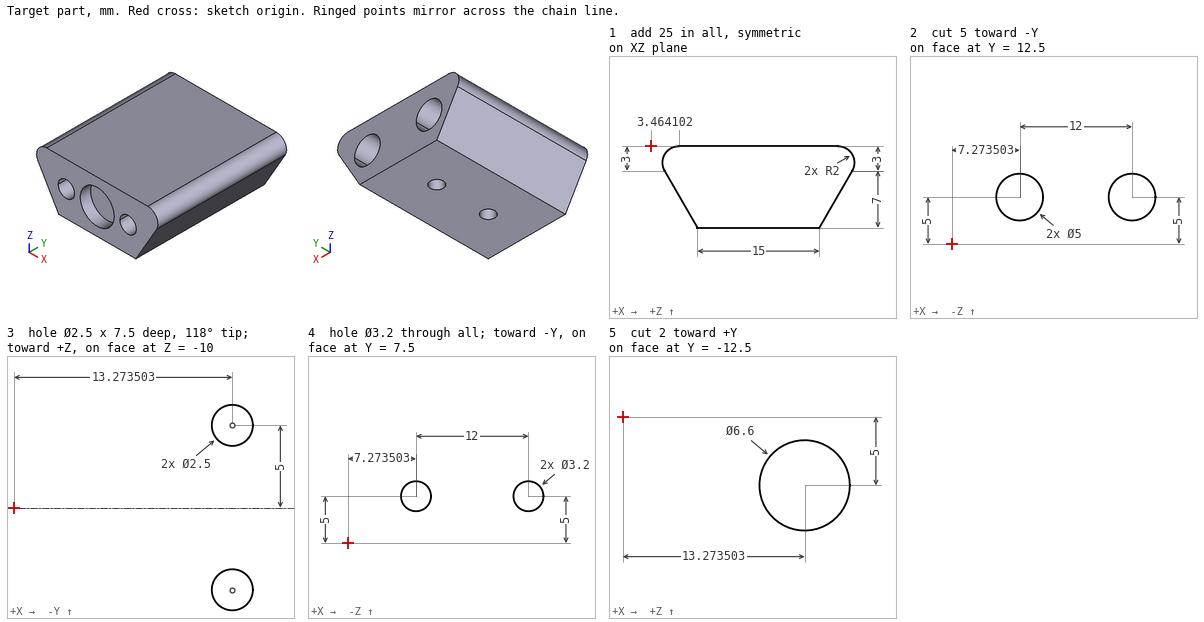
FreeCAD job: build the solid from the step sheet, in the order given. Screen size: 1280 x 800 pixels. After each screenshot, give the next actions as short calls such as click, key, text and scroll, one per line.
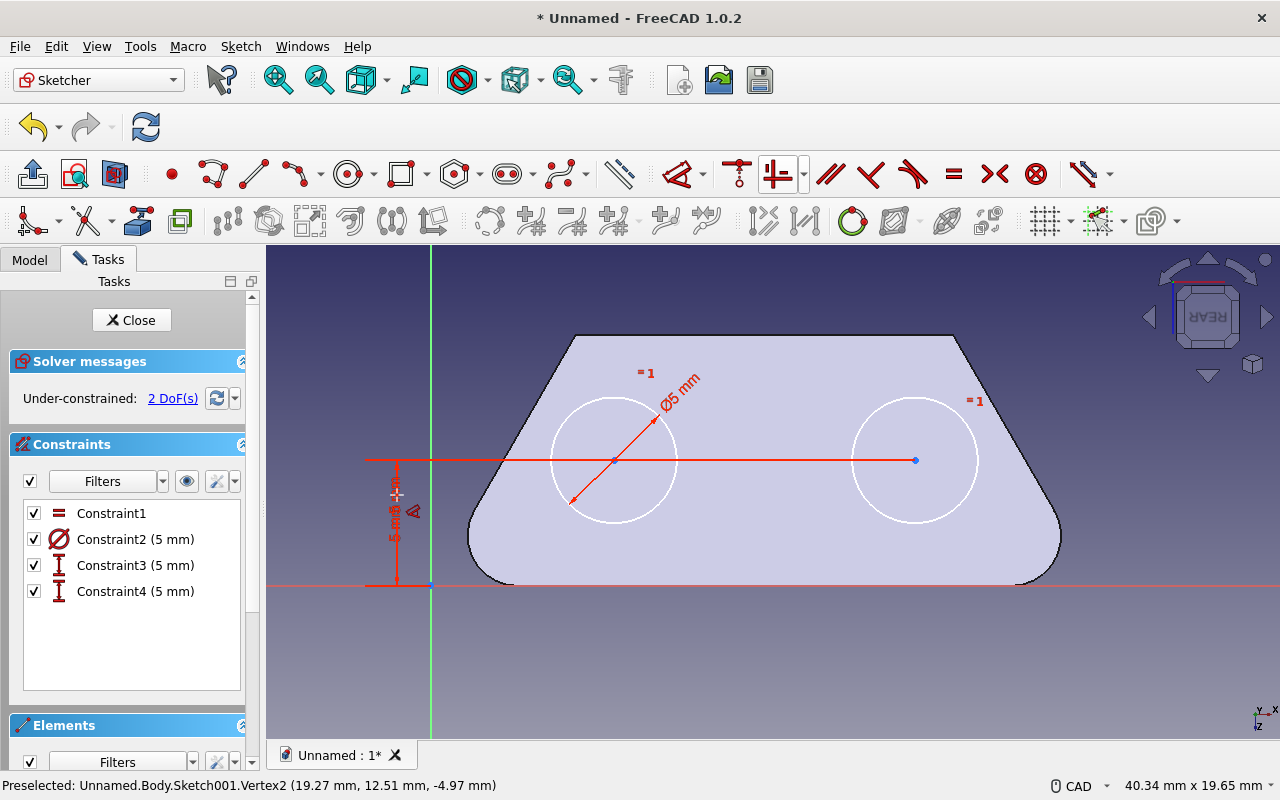
click(614, 460)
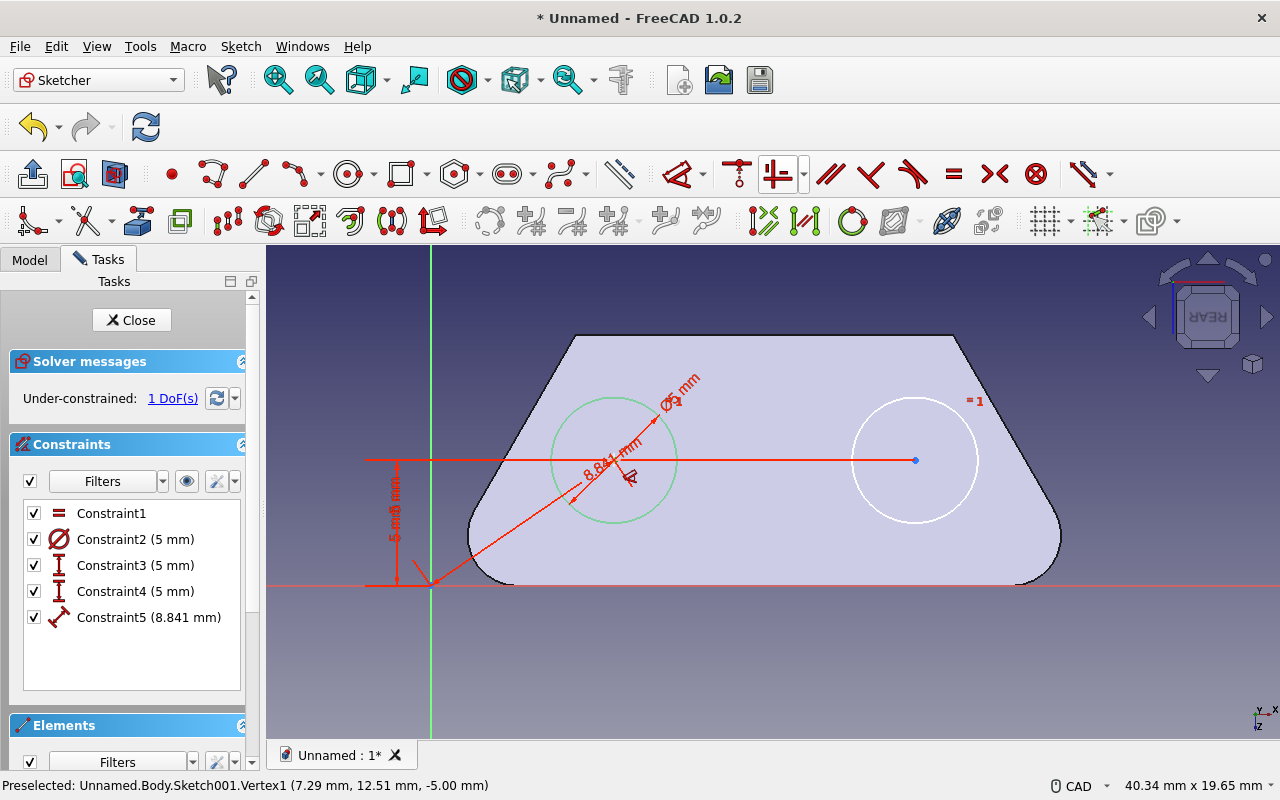
click(915, 460)
click(764, 426)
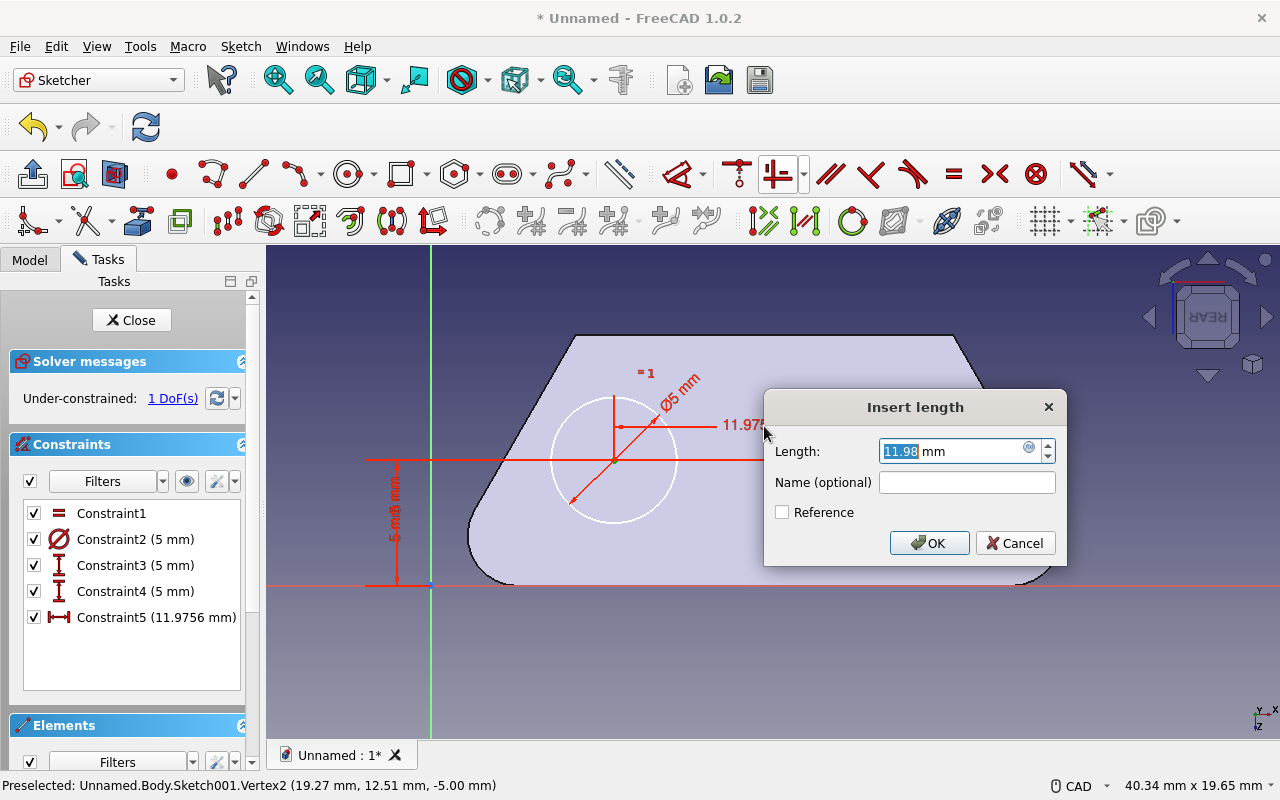
text(12)
key(Return)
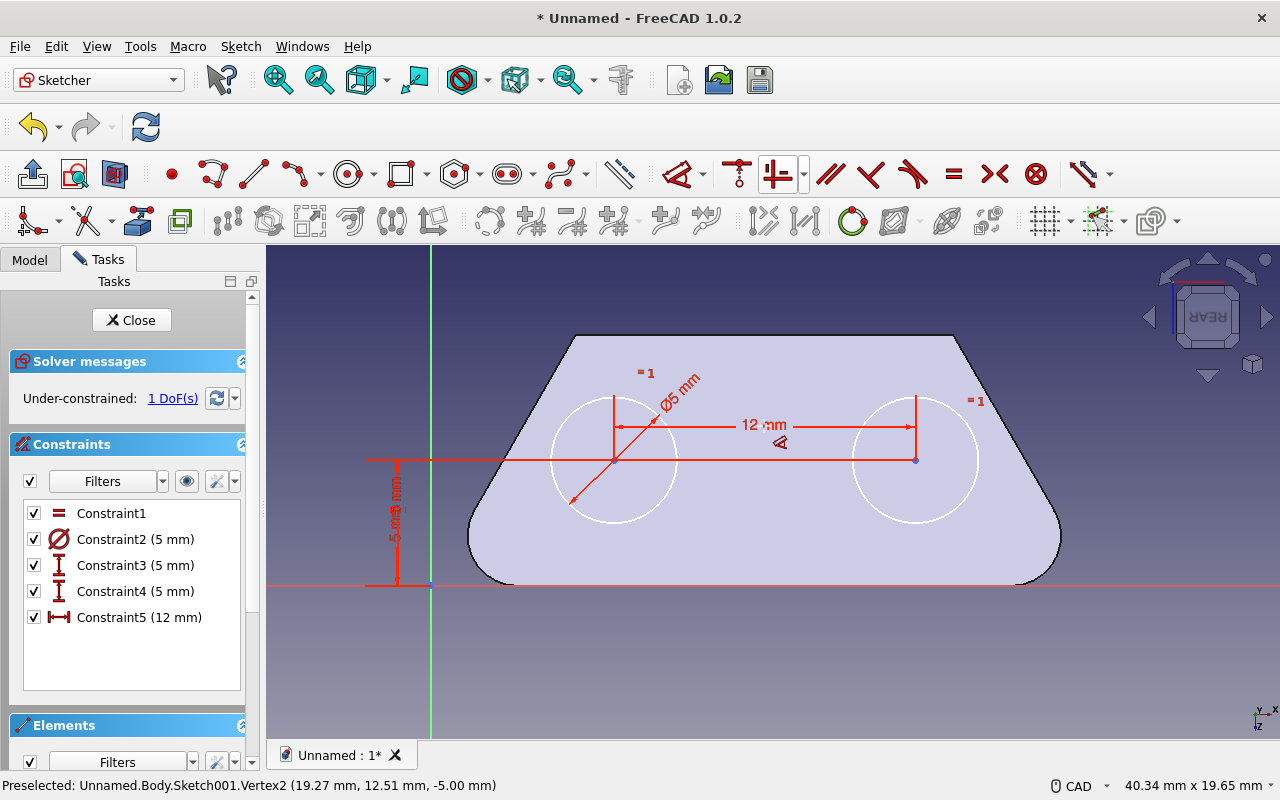
click(614, 460)
click(522, 620)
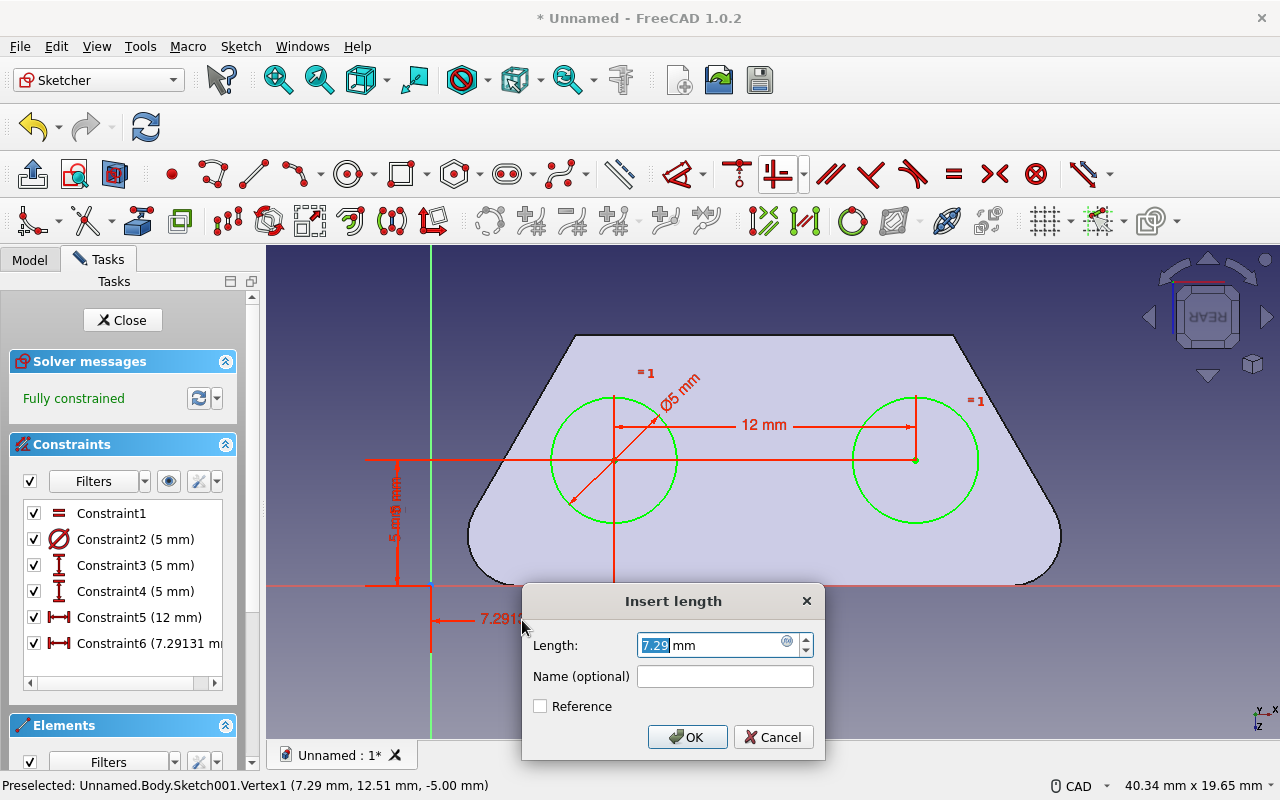
text(7.273503)
key(Return)
key(Escape)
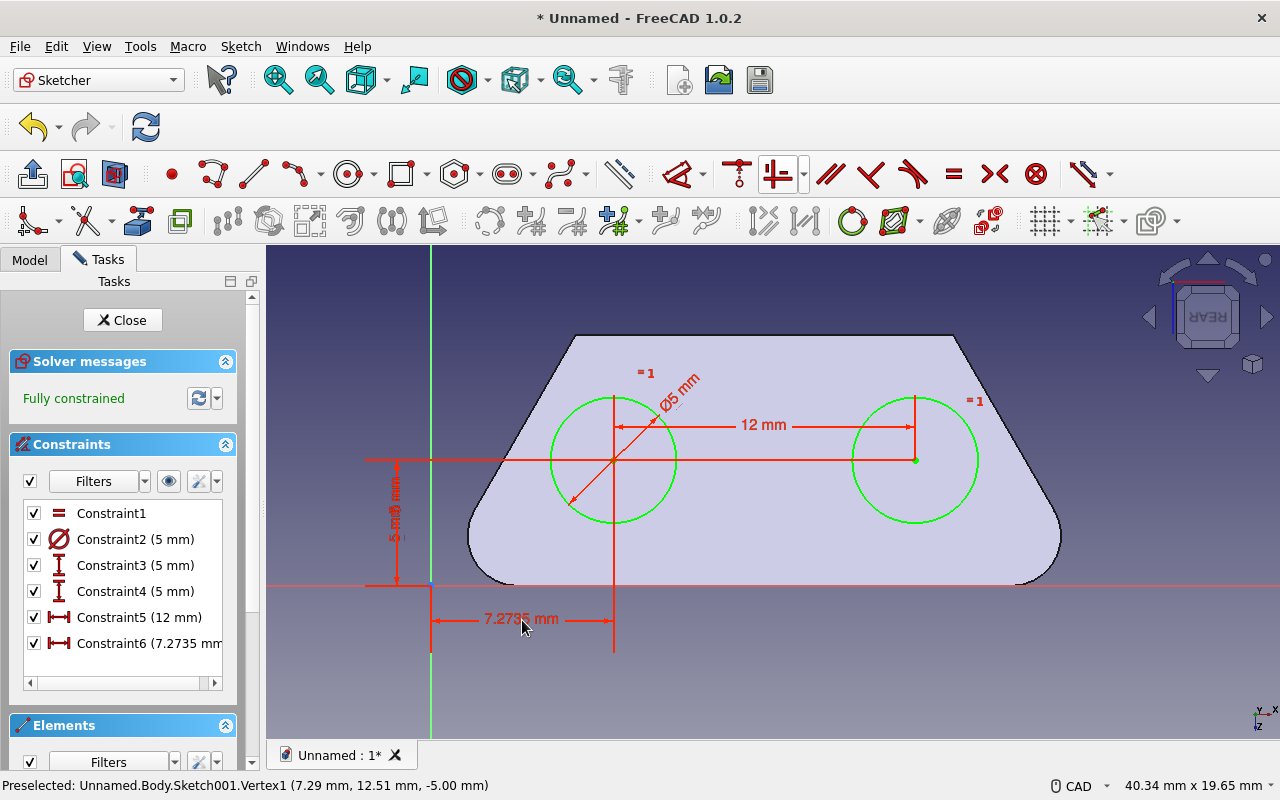
click(123, 320)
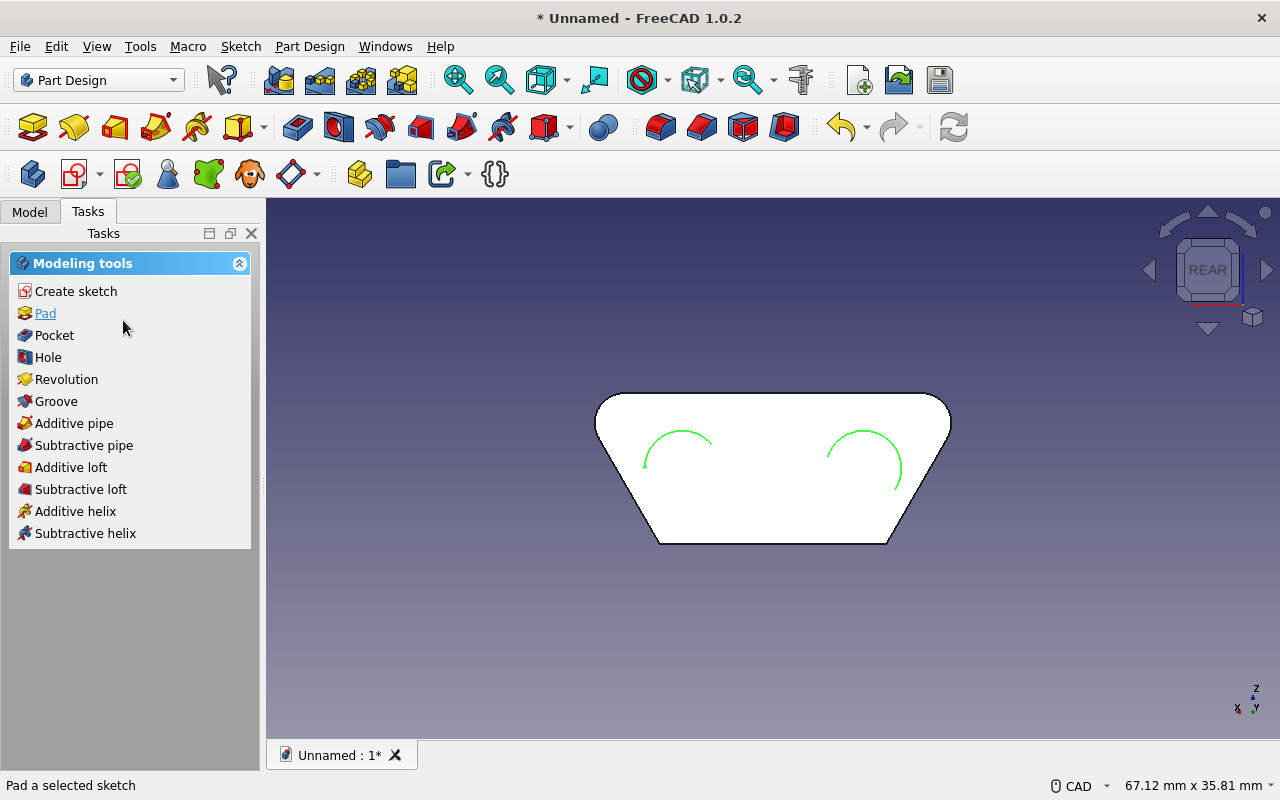
click(298, 128)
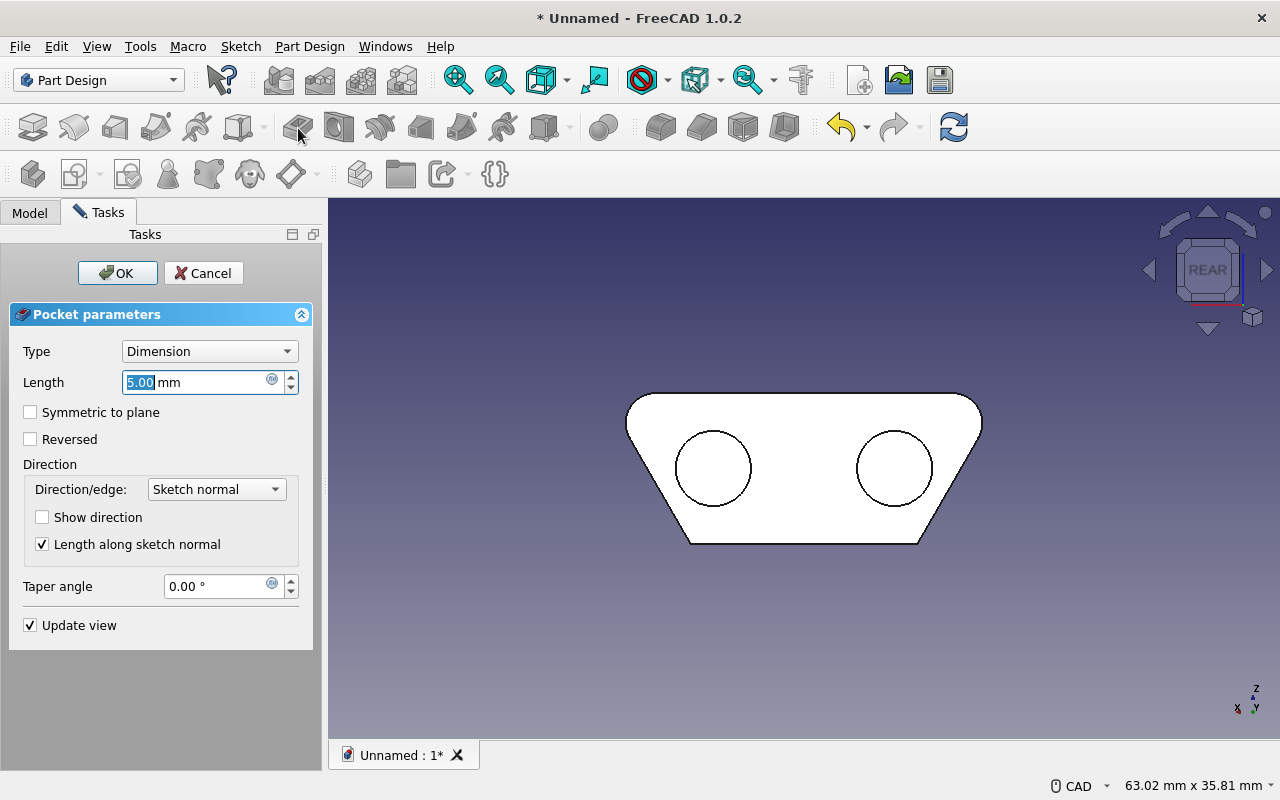
text(5)
key(Tab)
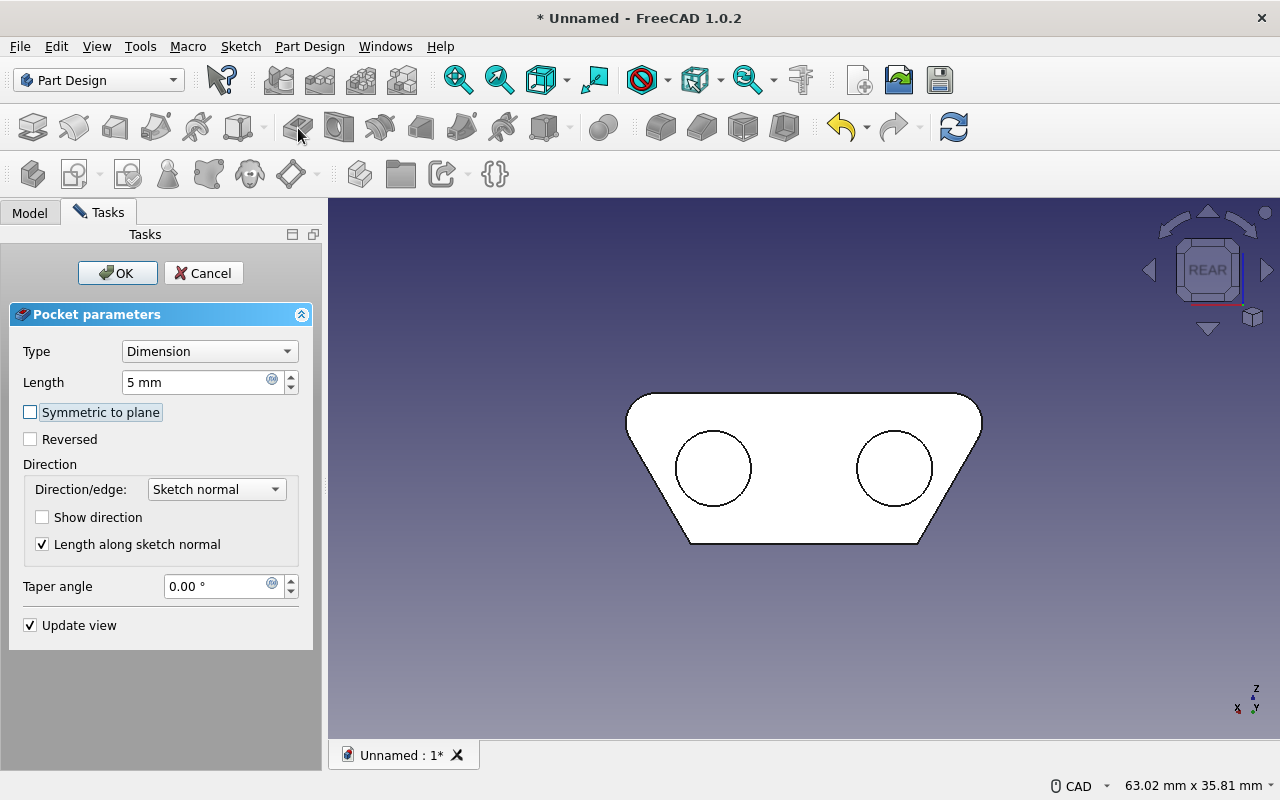
click(118, 273)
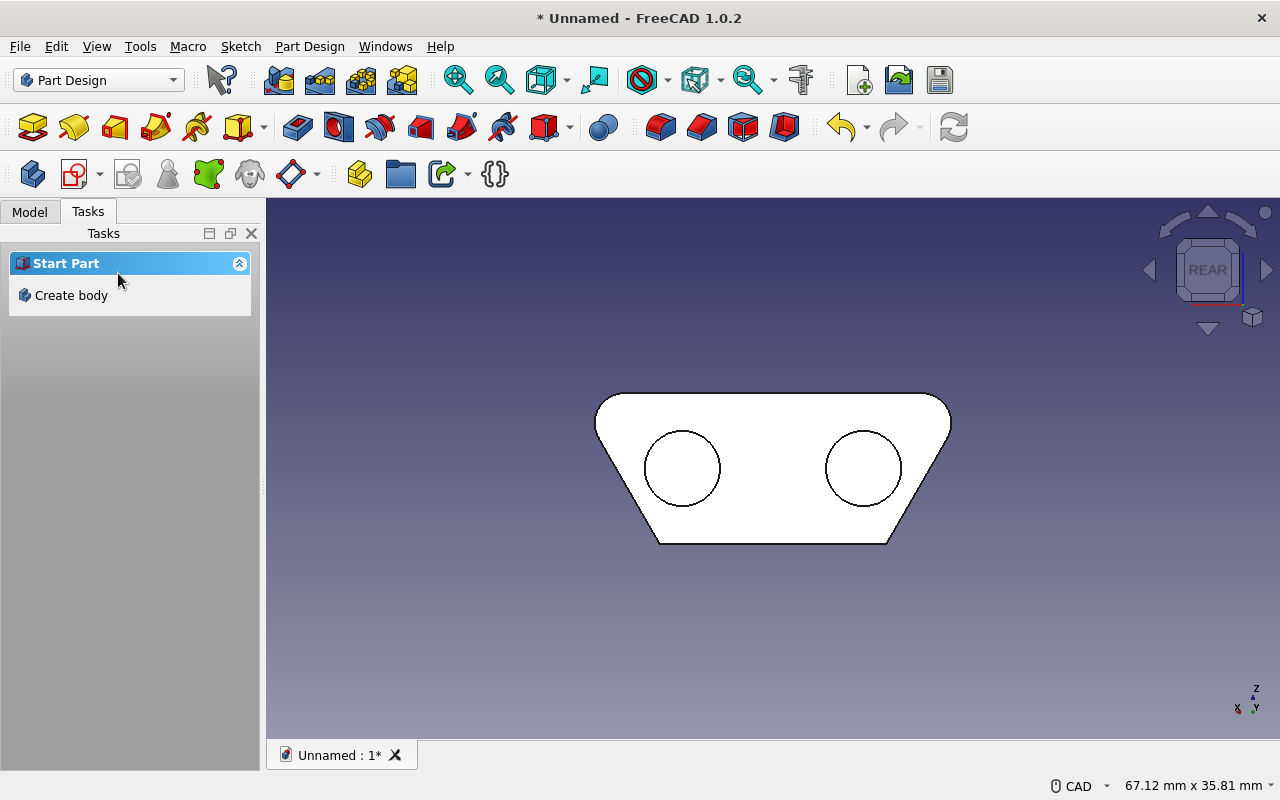
click(459, 80)